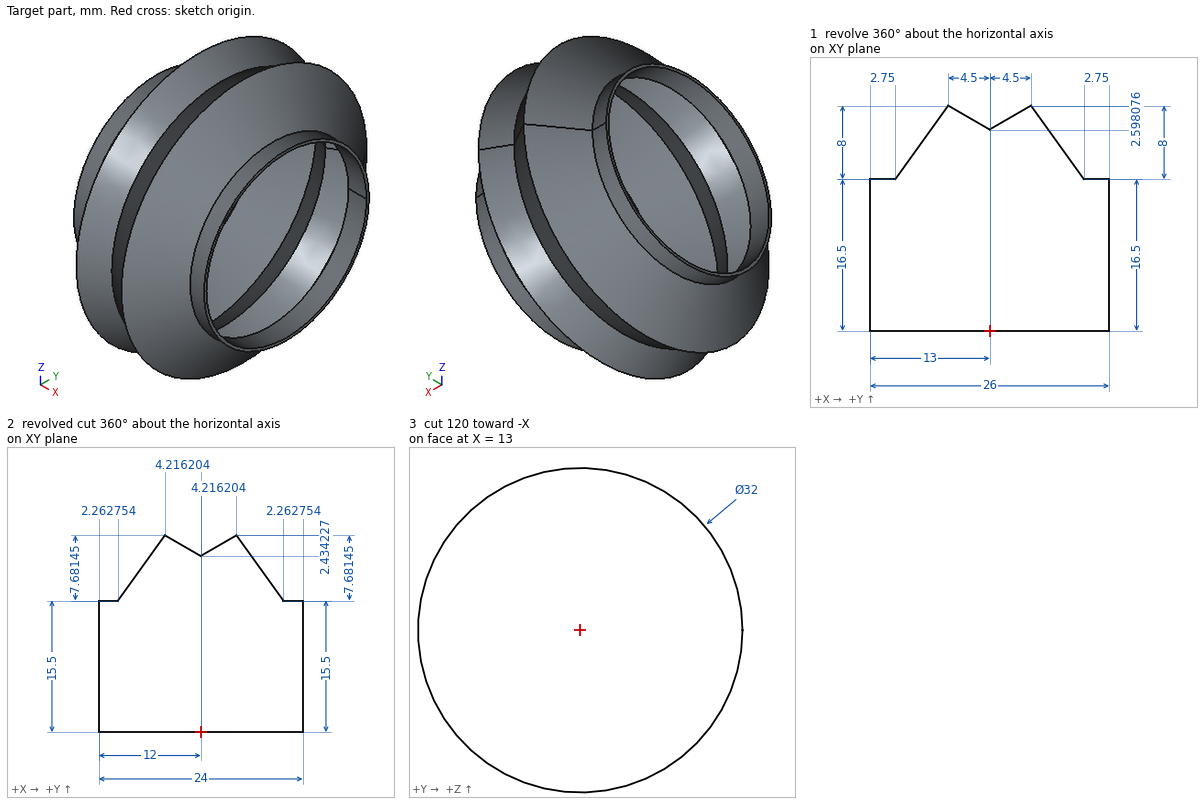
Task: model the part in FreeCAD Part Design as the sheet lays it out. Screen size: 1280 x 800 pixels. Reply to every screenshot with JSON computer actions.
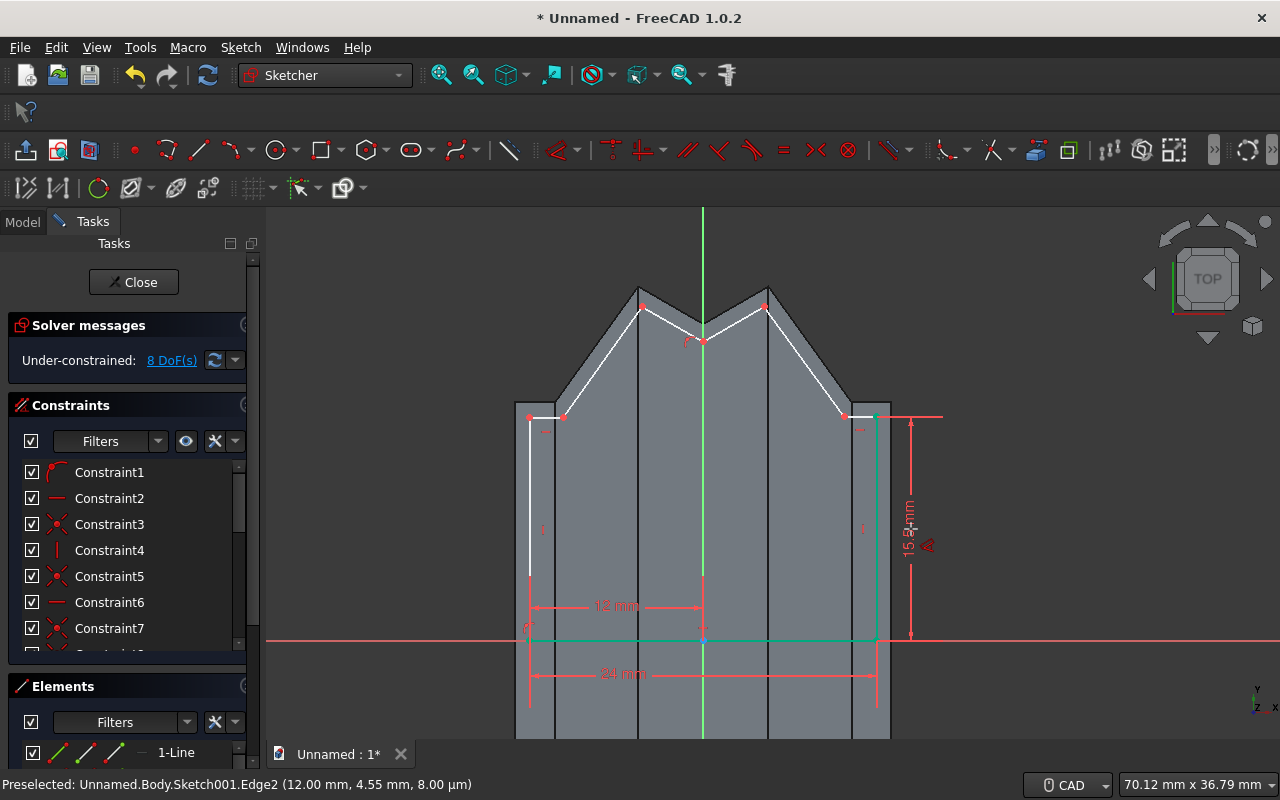
{"action": "left_click", "coordinate": [530, 485]}
{"action": "left_click", "coordinate": [496, 529]}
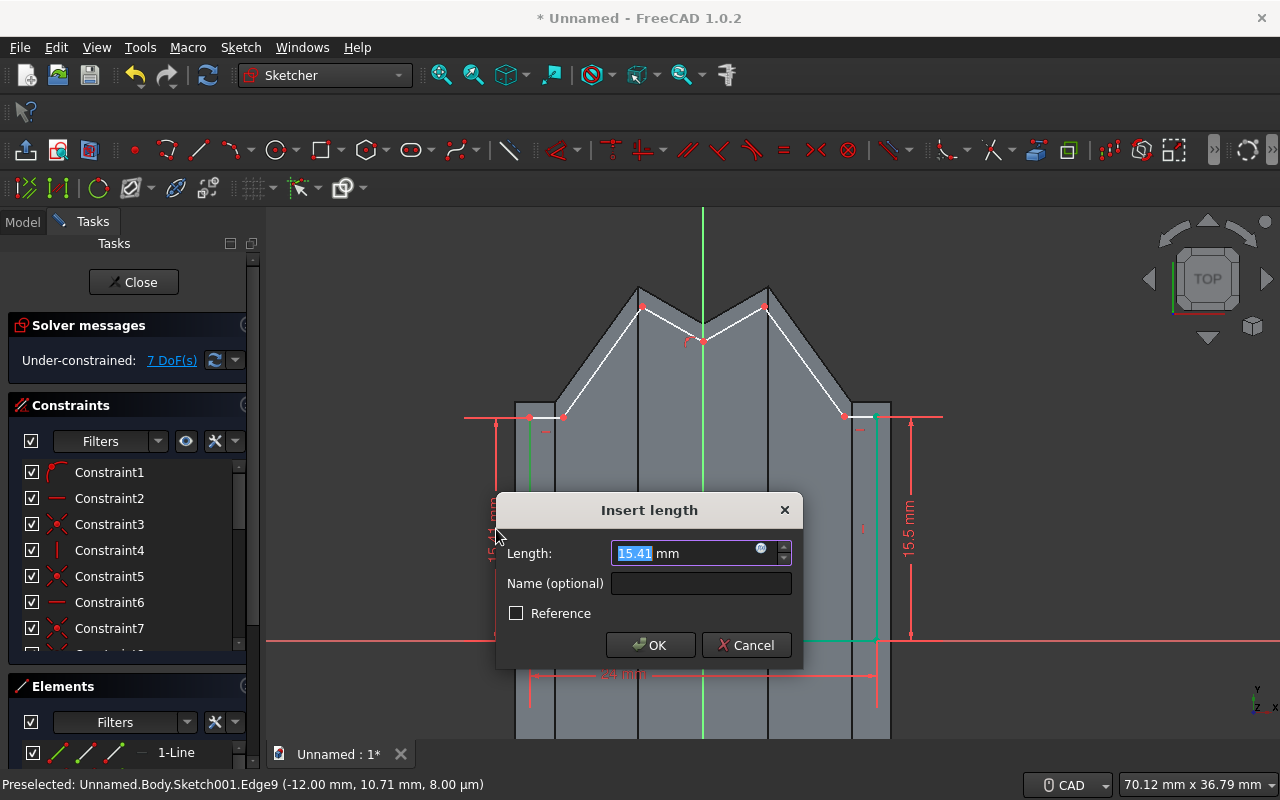
{"action": "type", "text": "15.5"}
{"action": "key", "text": "Return"}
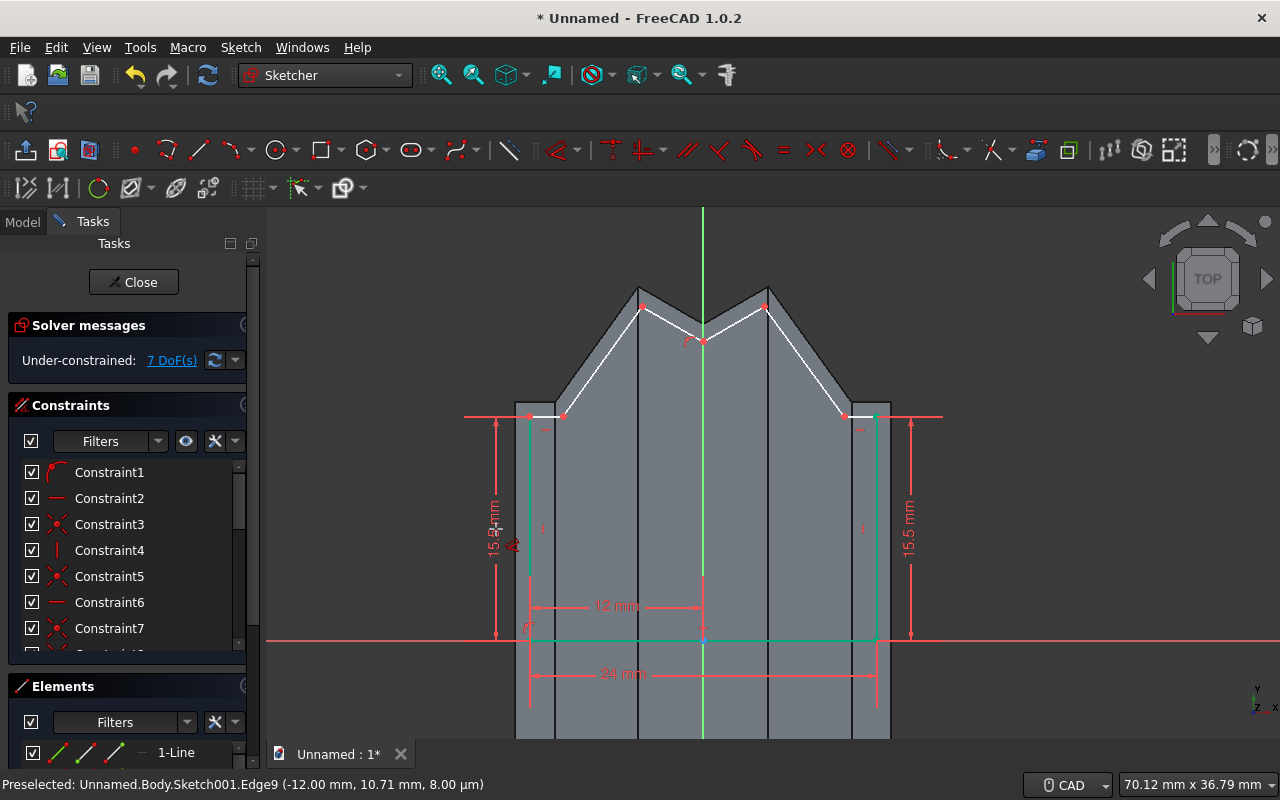
{"action": "scroll", "coordinate": [867, 417], "scroll_direction": "up", "scroll_amount": 2}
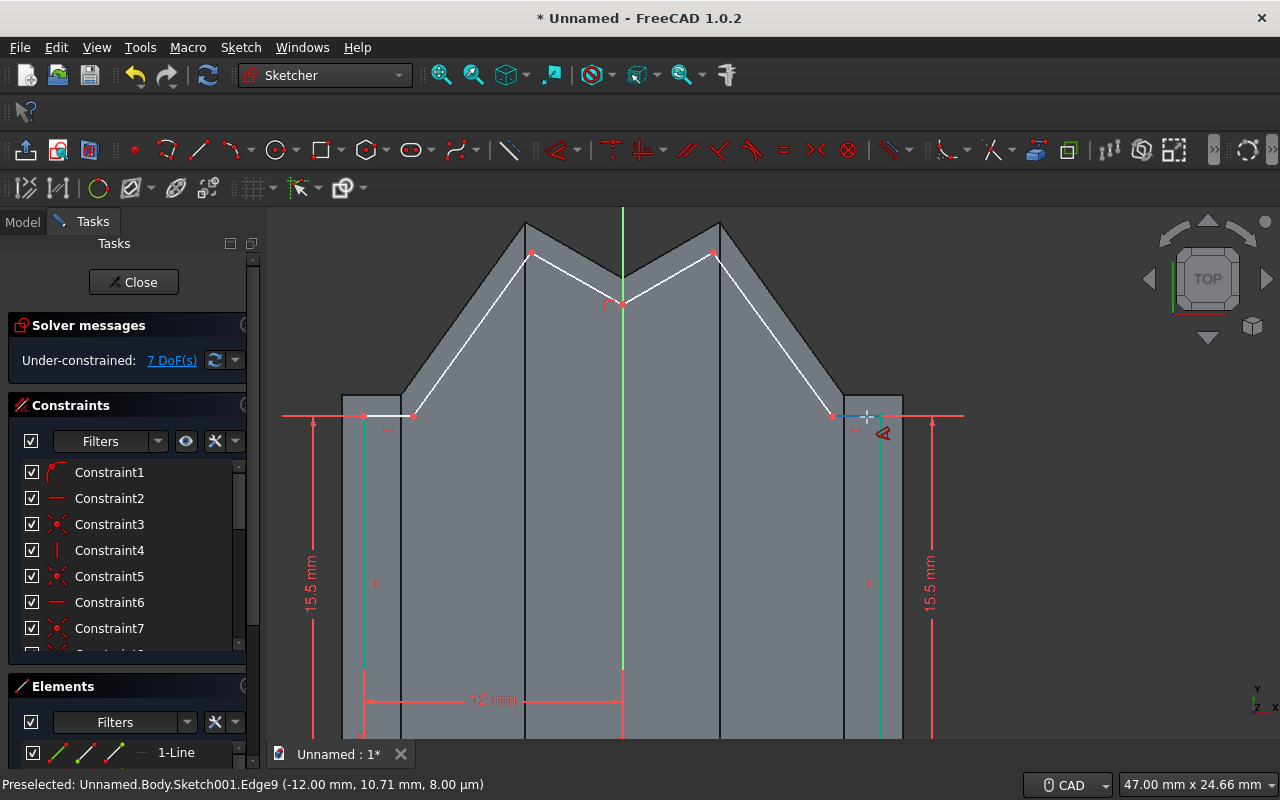
{"action": "left_click", "coordinate": [867, 416]}
{"action": "left_click", "coordinate": [857, 382]}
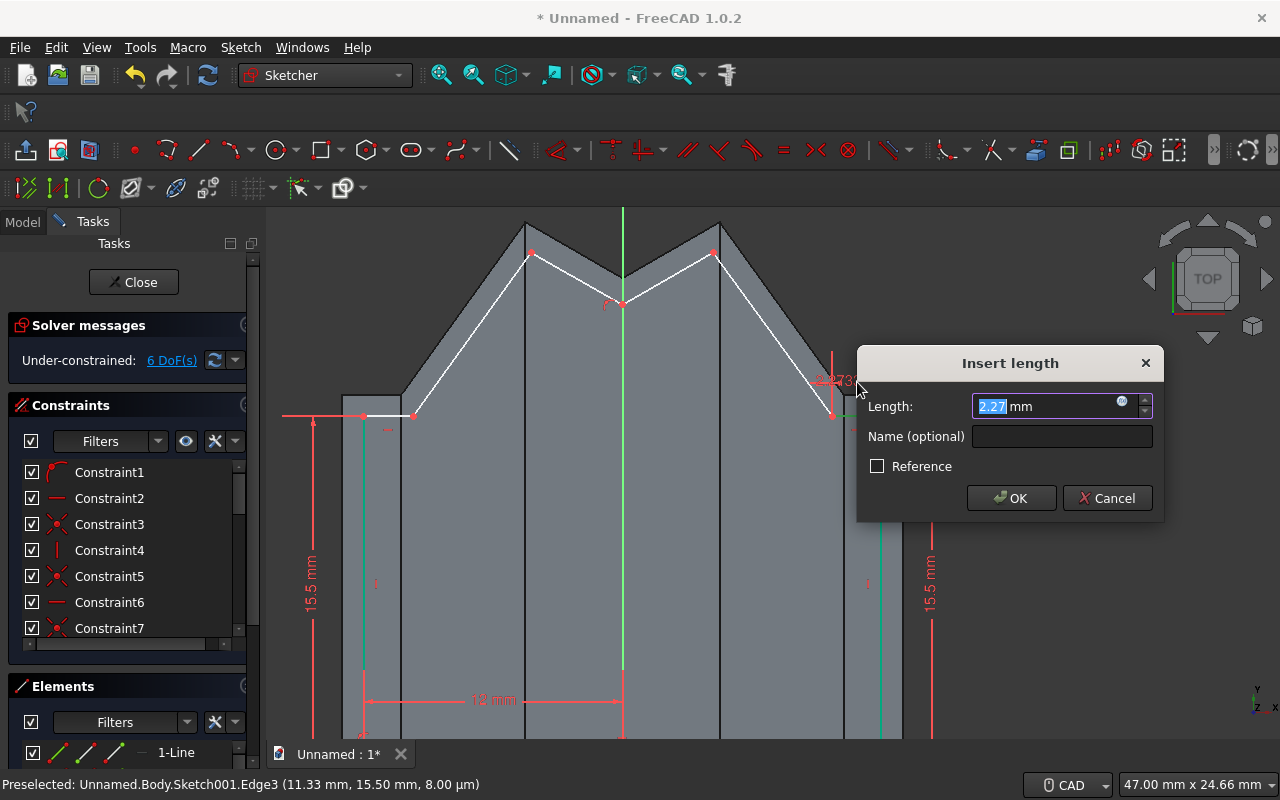
{"action": "type", "text": "2.262754"}
{"action": "key", "text": "Return"}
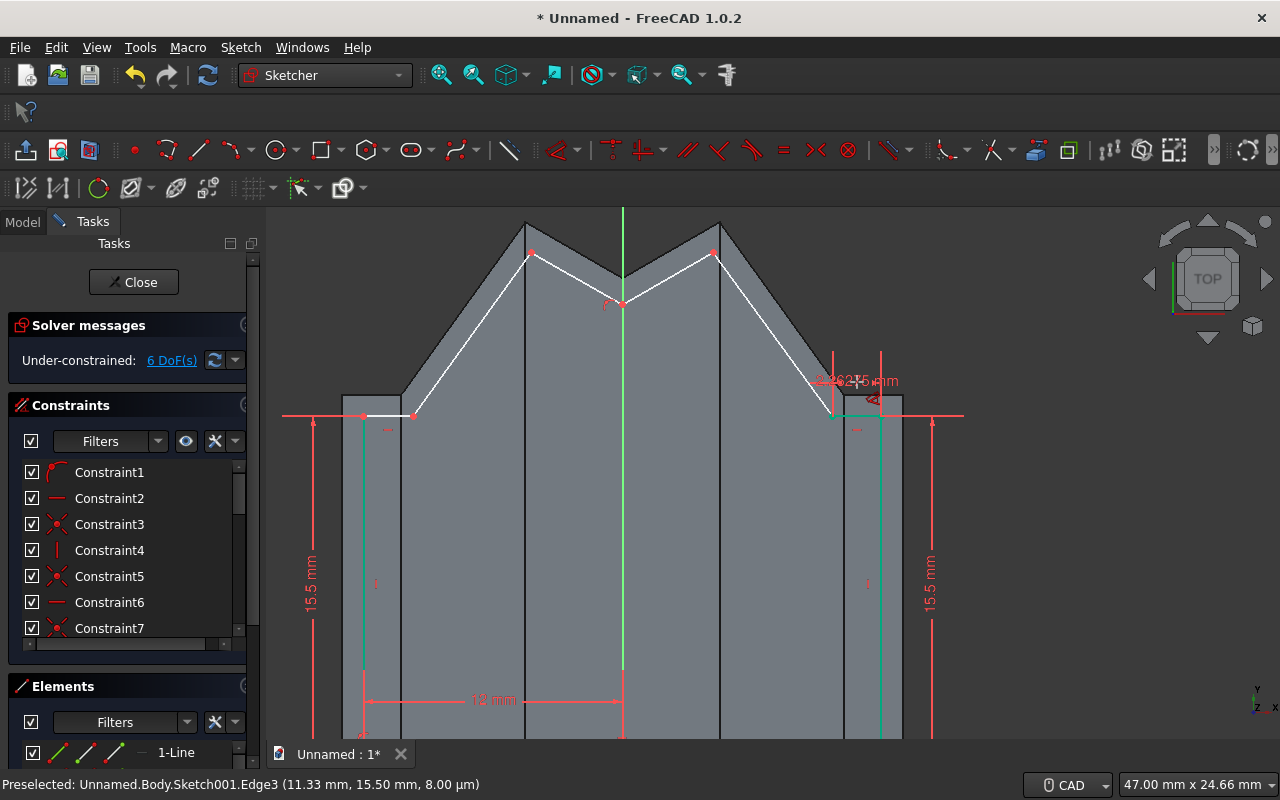
{"action": "left_click", "coordinate": [398, 416]}
{"action": "left_click", "coordinate": [388, 382]}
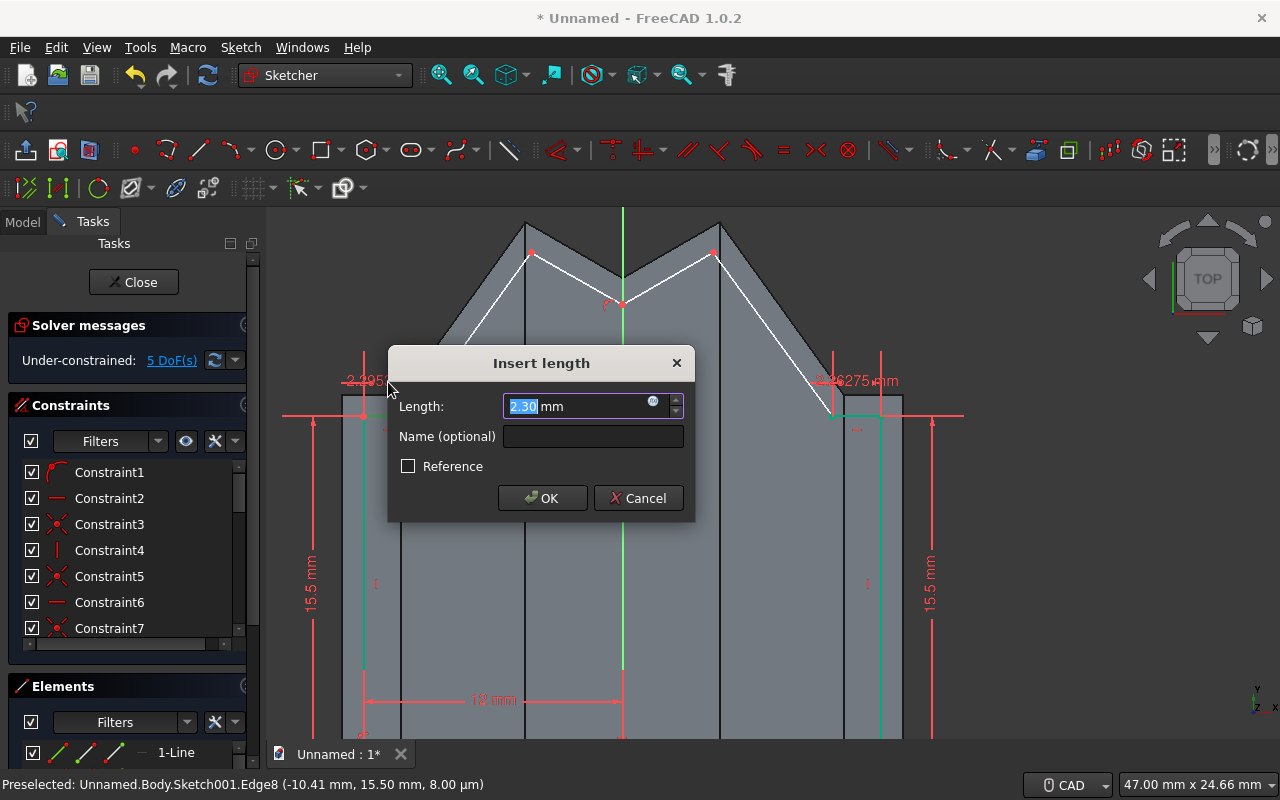
{"action": "type", "text": "2.262754"}
{"action": "key", "text": "Return"}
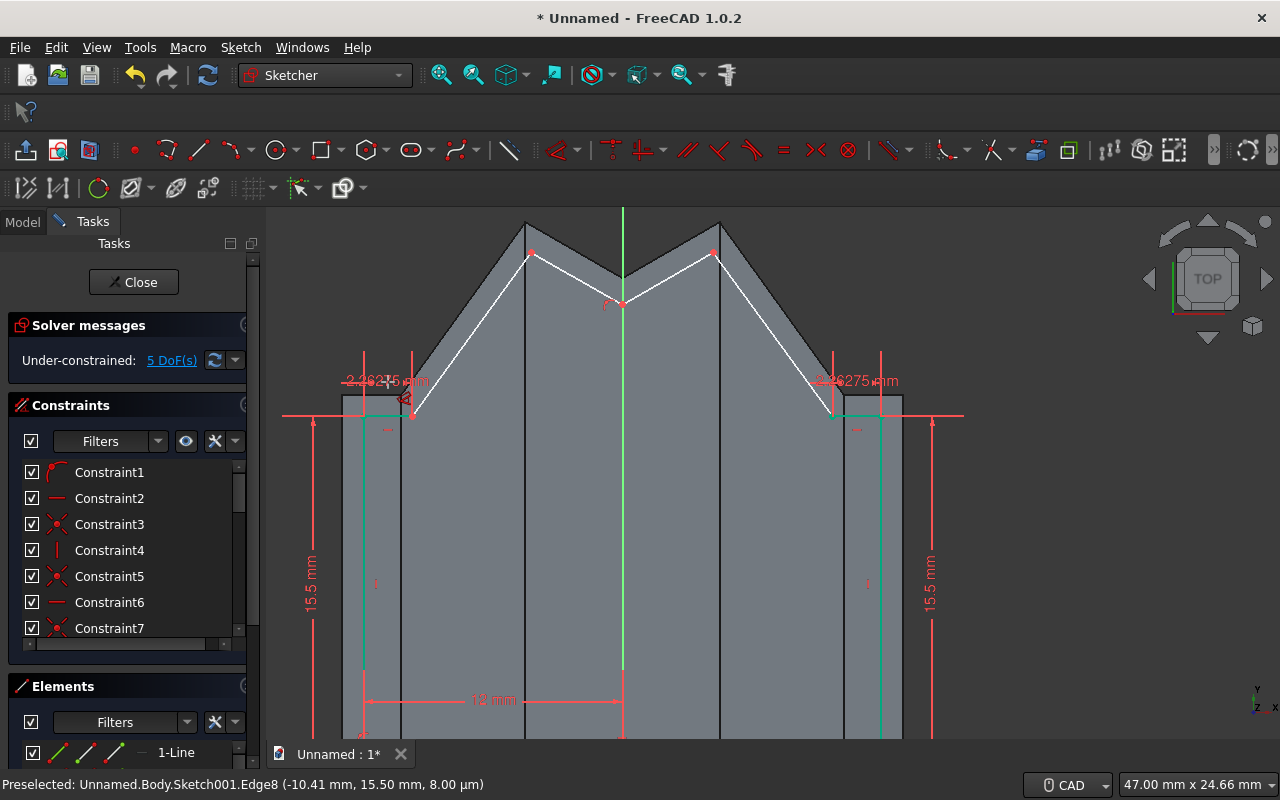
{"action": "left_click", "coordinate": [797, 367]}
{"action": "left_click", "coordinate": [867, 335]}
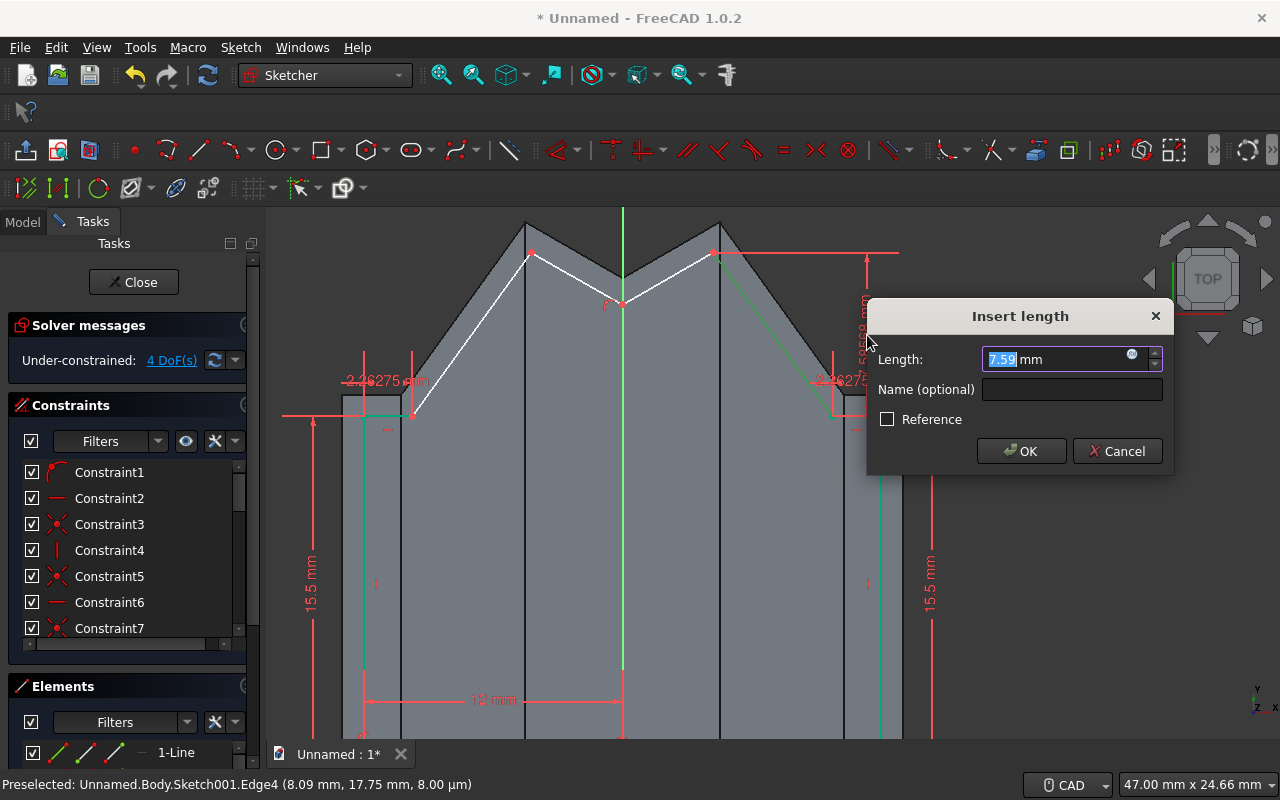
{"action": "type", "text": "7.68145"}
{"action": "key", "text": "Return"}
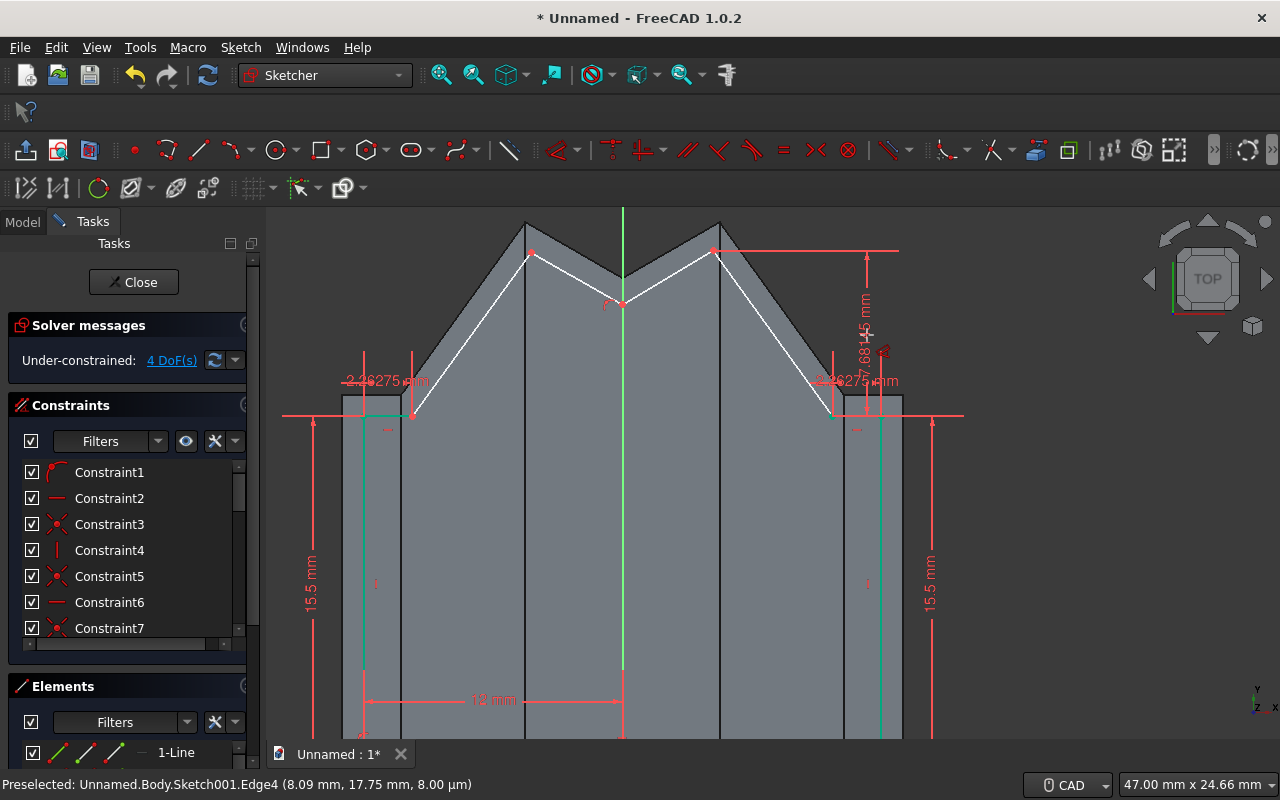
{"action": "left_click", "coordinate": [495, 302]}
{"action": "left_click", "coordinate": [378, 335]}